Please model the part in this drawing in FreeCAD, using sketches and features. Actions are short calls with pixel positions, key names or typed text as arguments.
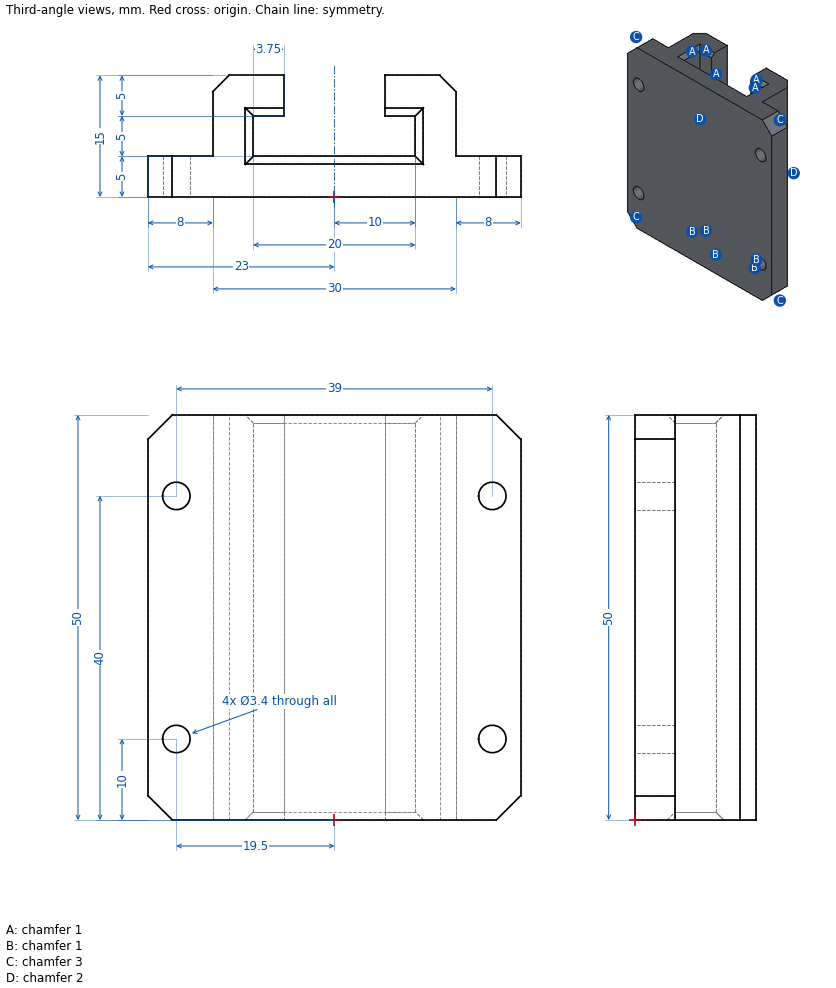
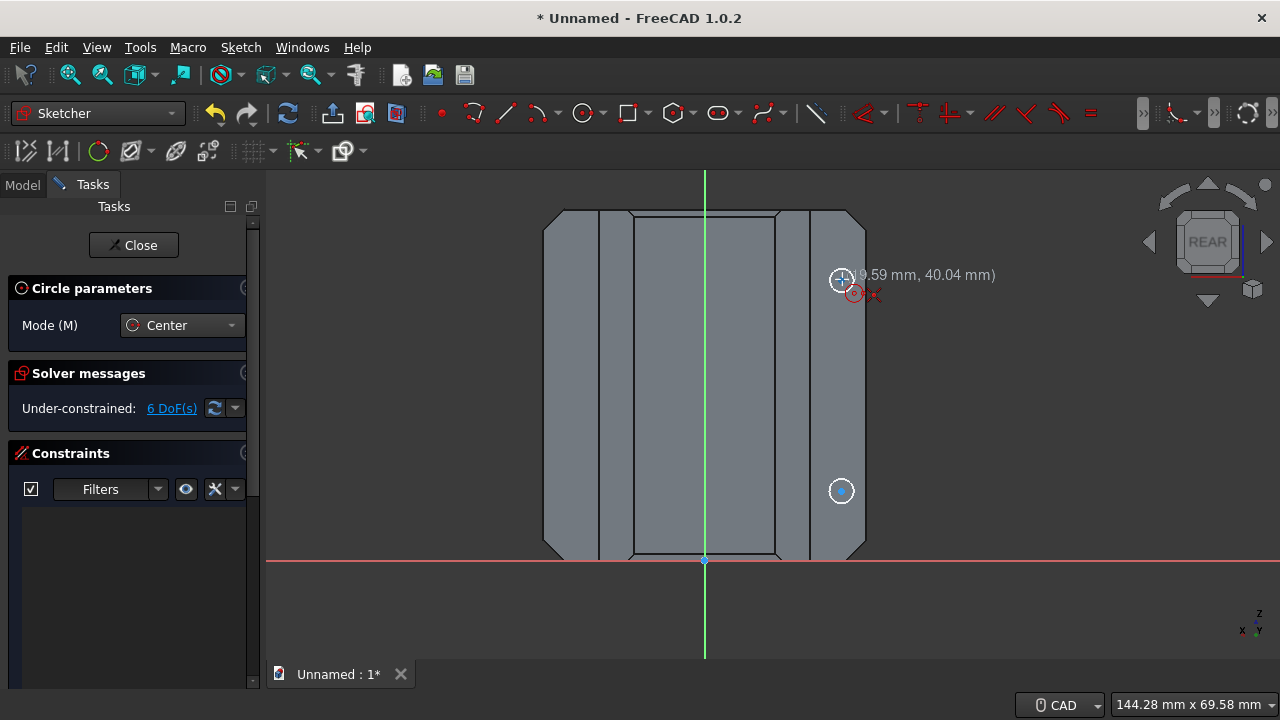
scroll(568, 280, up, 4)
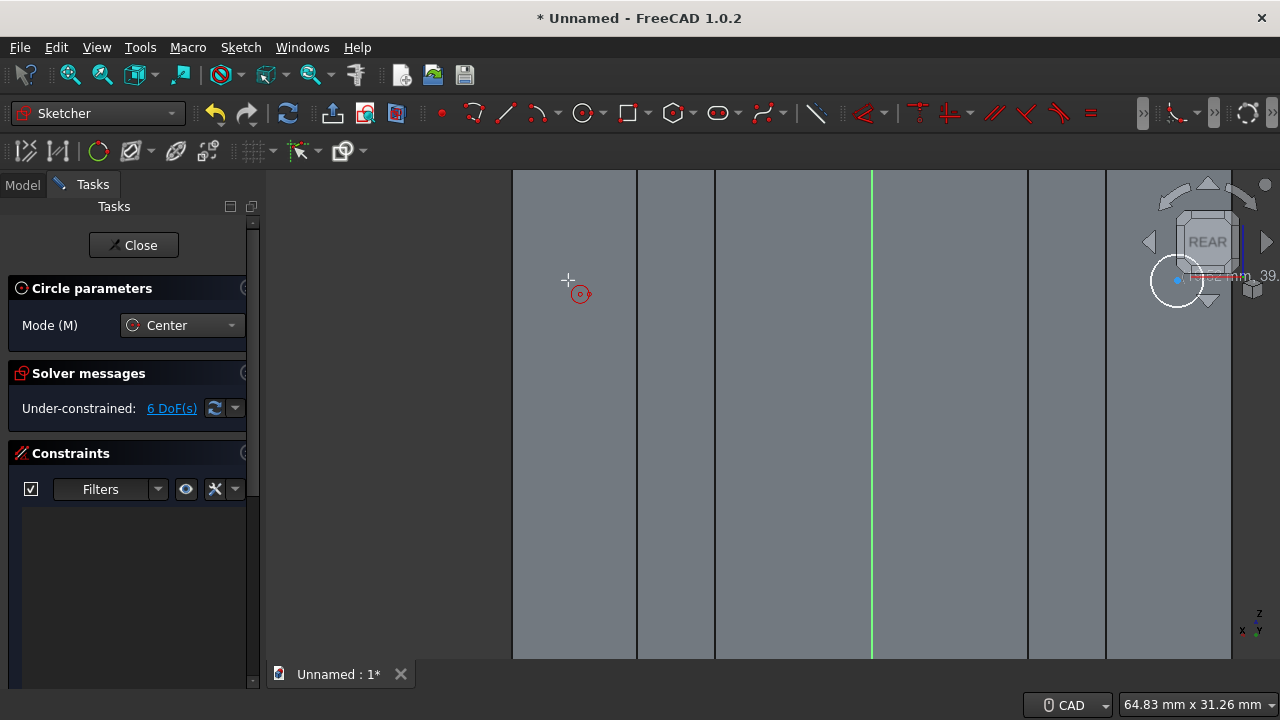
click(567, 279)
click(586, 261)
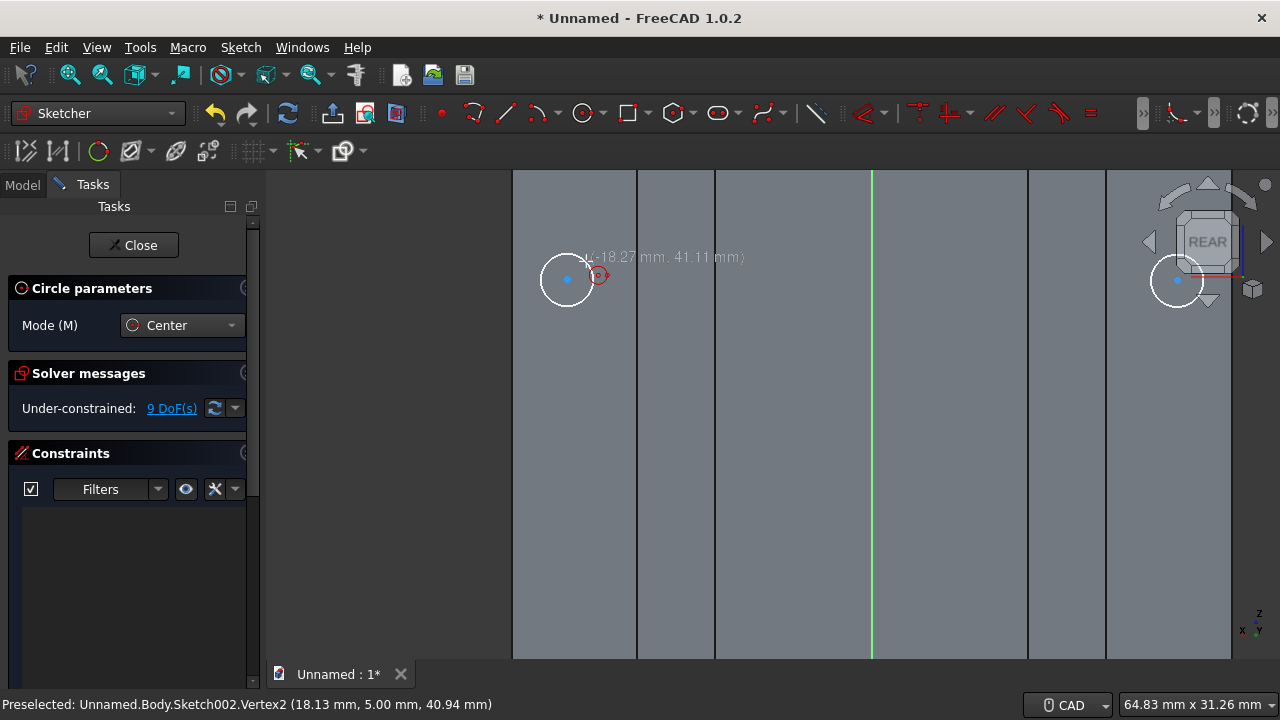
scroll(568, 280, down, 4)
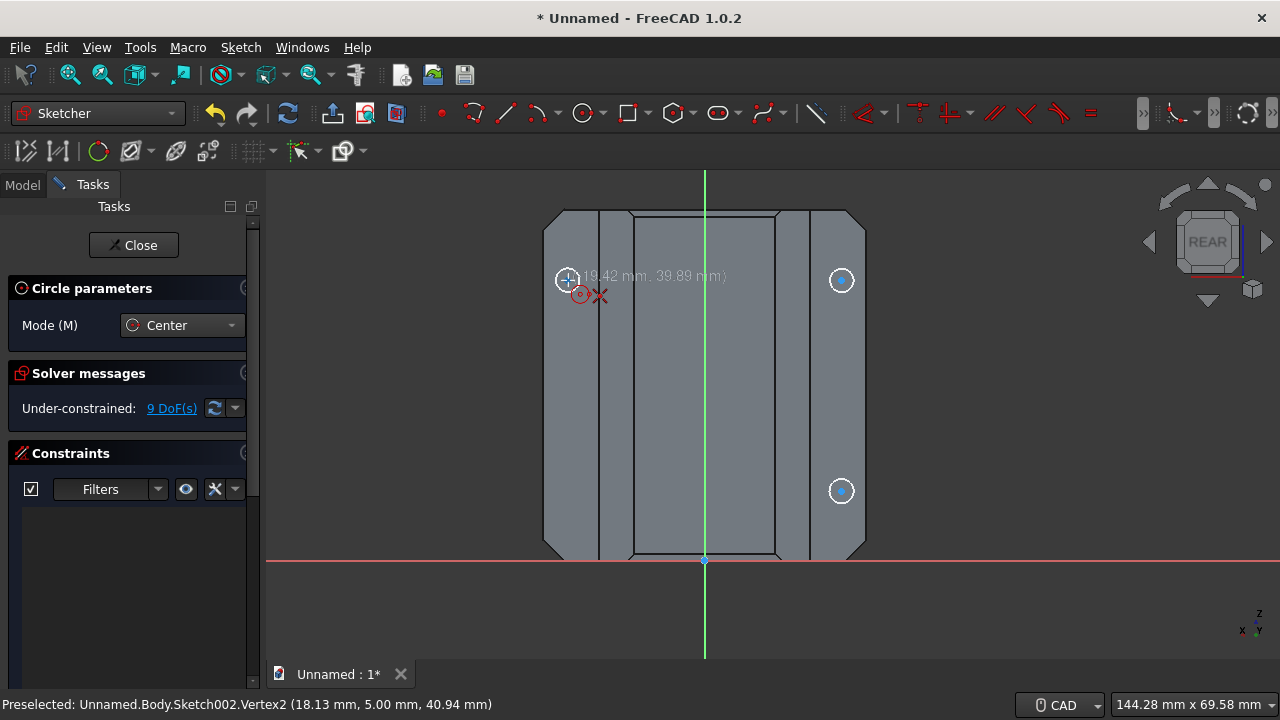
scroll(568, 491, up, 4)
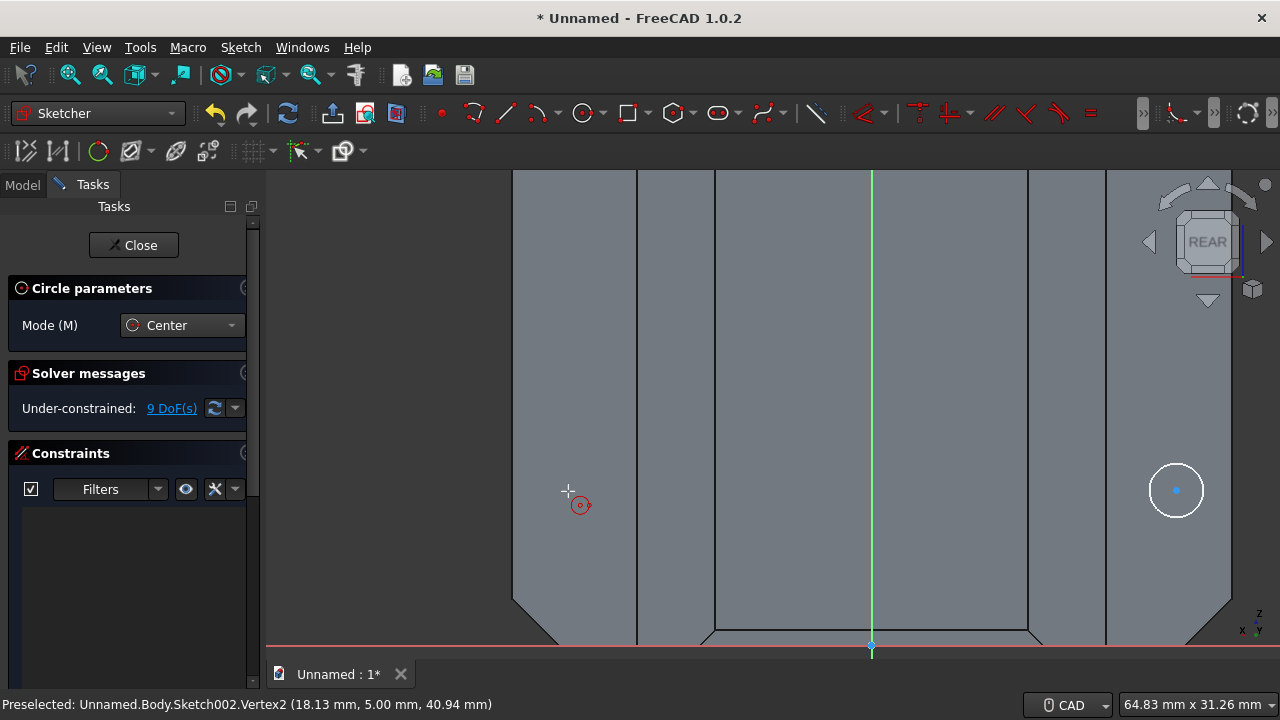
click(567, 489)
click(586, 471)
key(Escape)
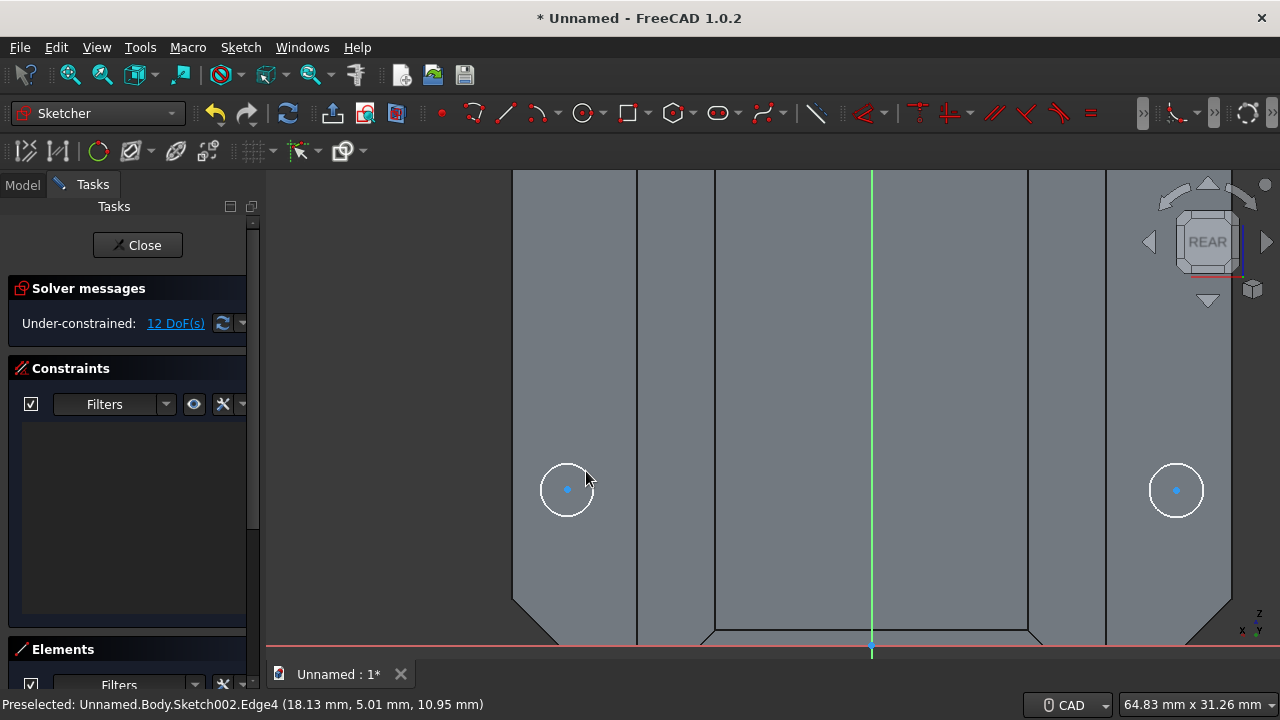
scroll(568, 492, down, 4)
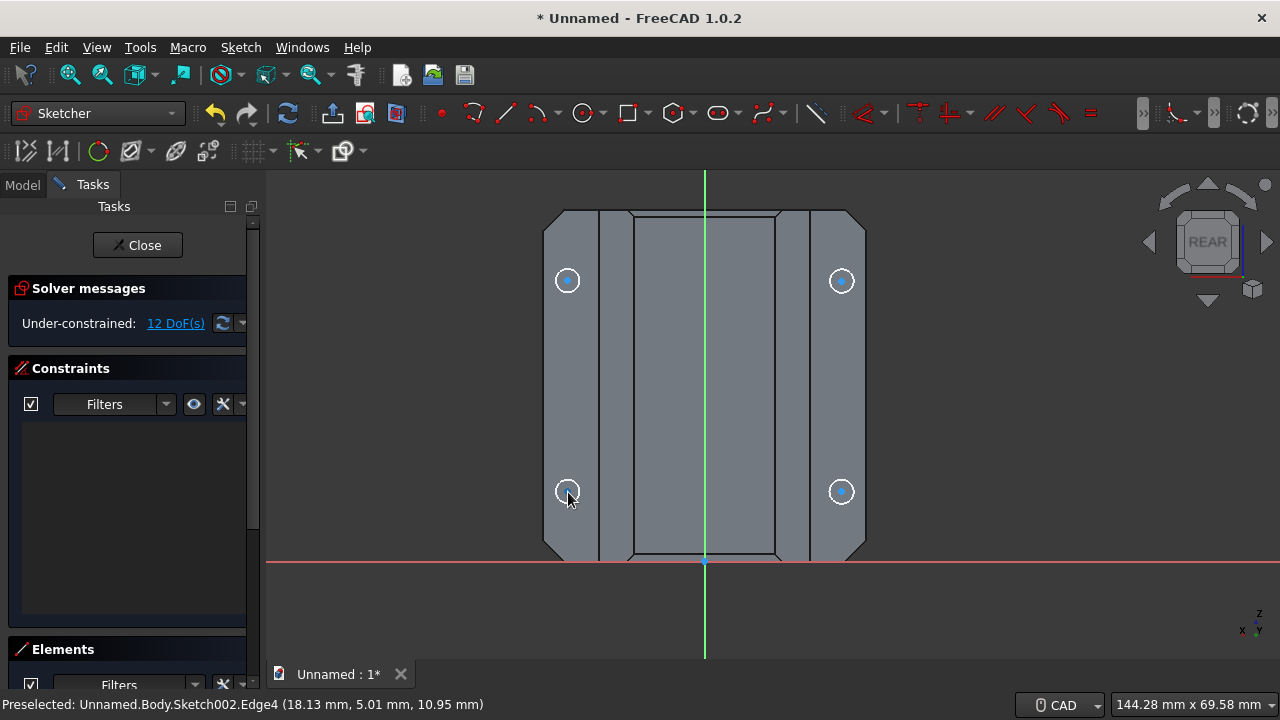
click(850, 483)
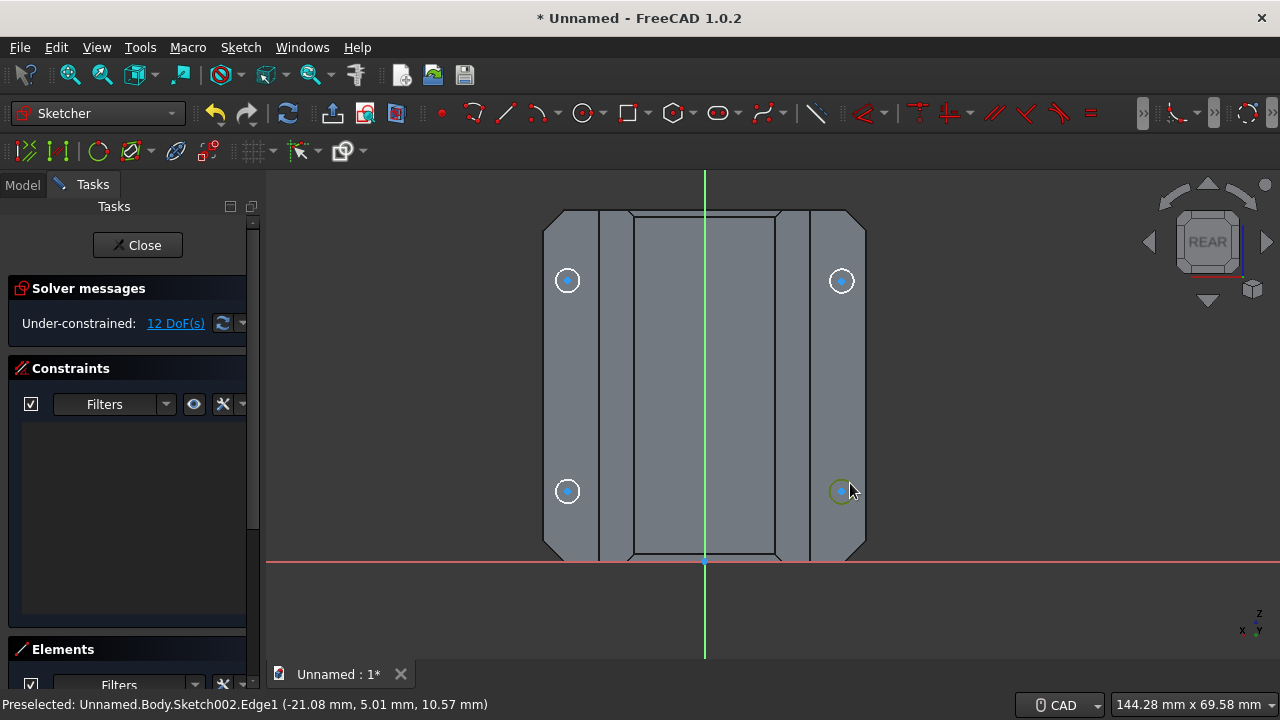
click(850, 273)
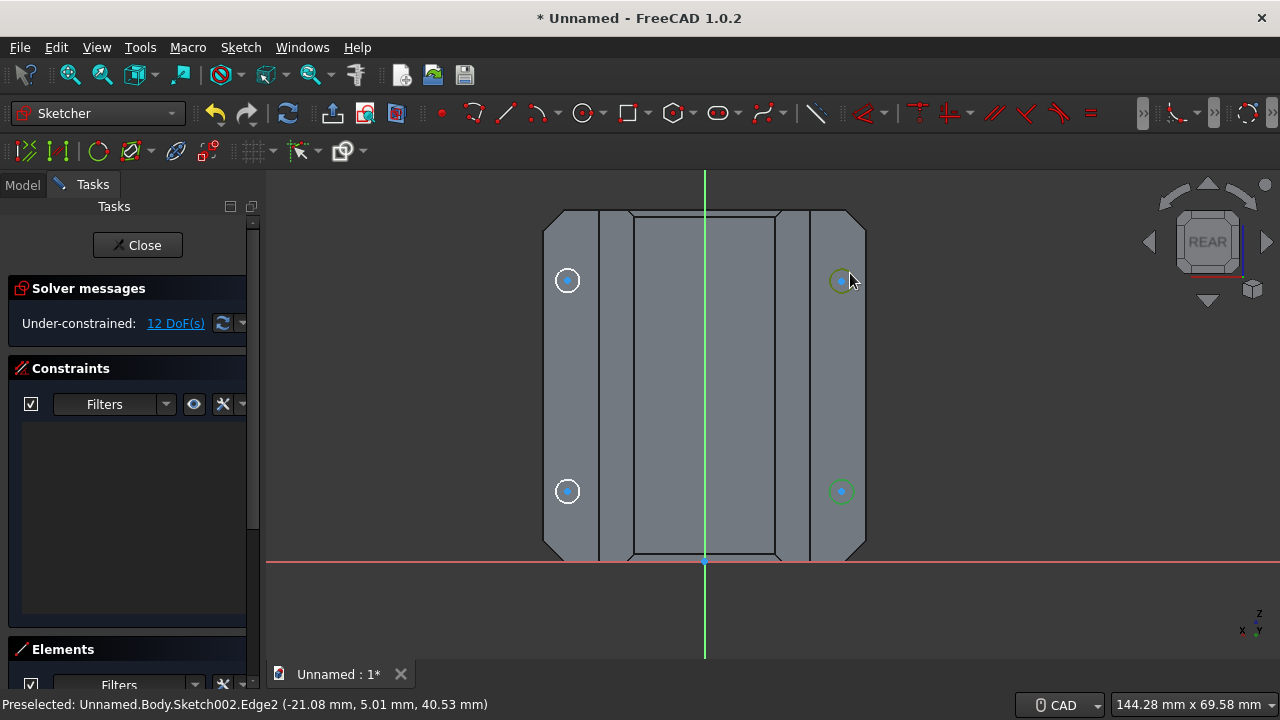
click(576, 272)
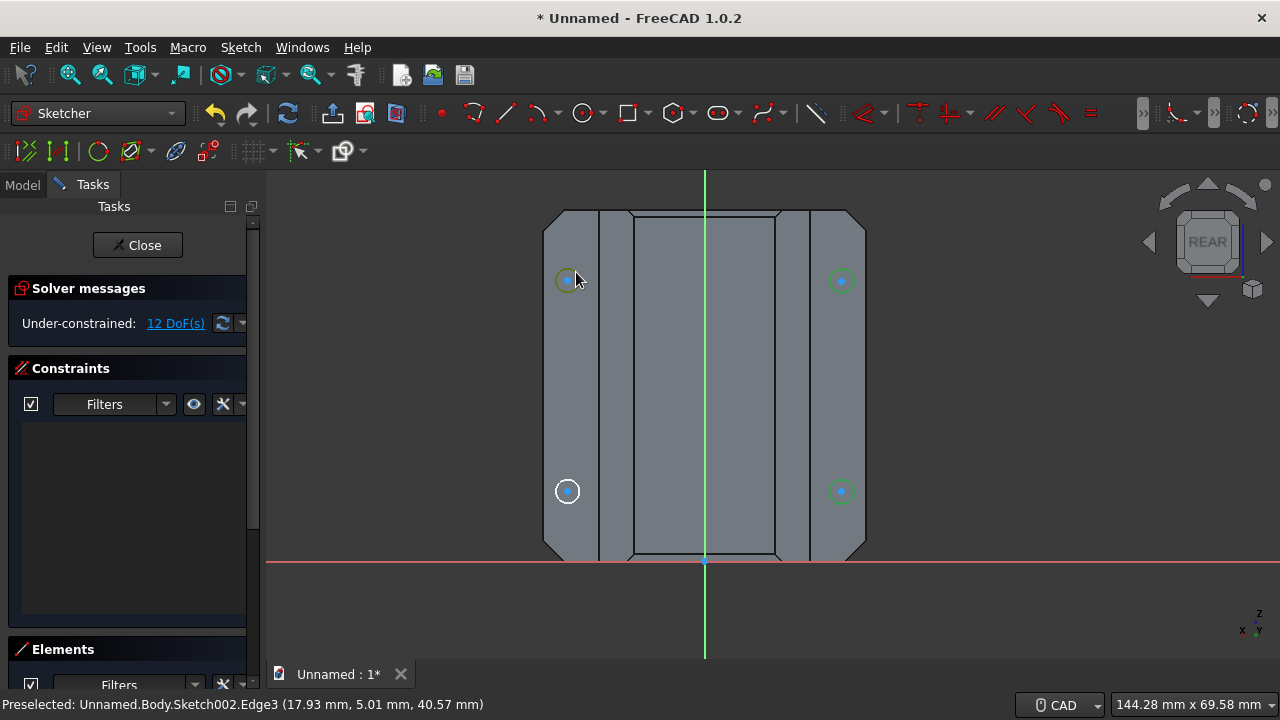
click(576, 483)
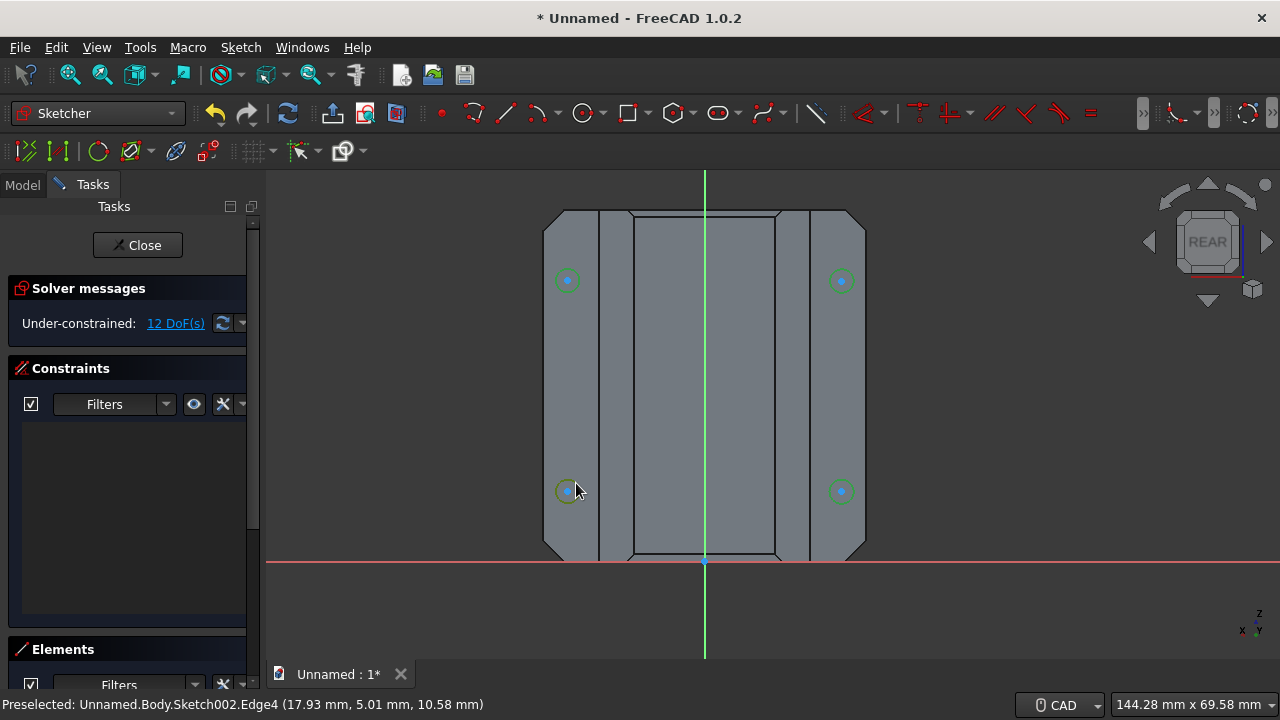
key(e)